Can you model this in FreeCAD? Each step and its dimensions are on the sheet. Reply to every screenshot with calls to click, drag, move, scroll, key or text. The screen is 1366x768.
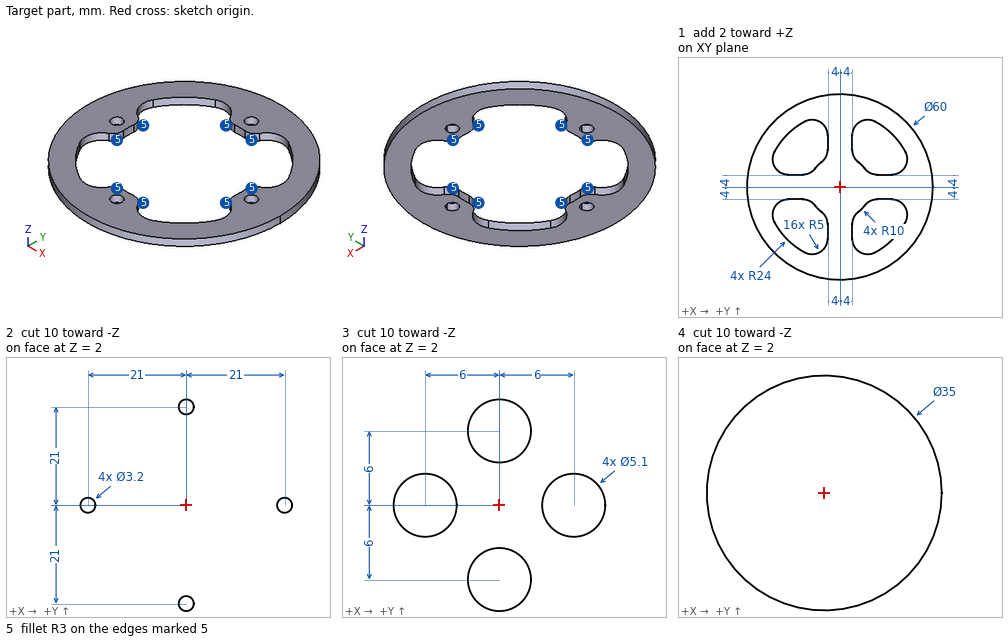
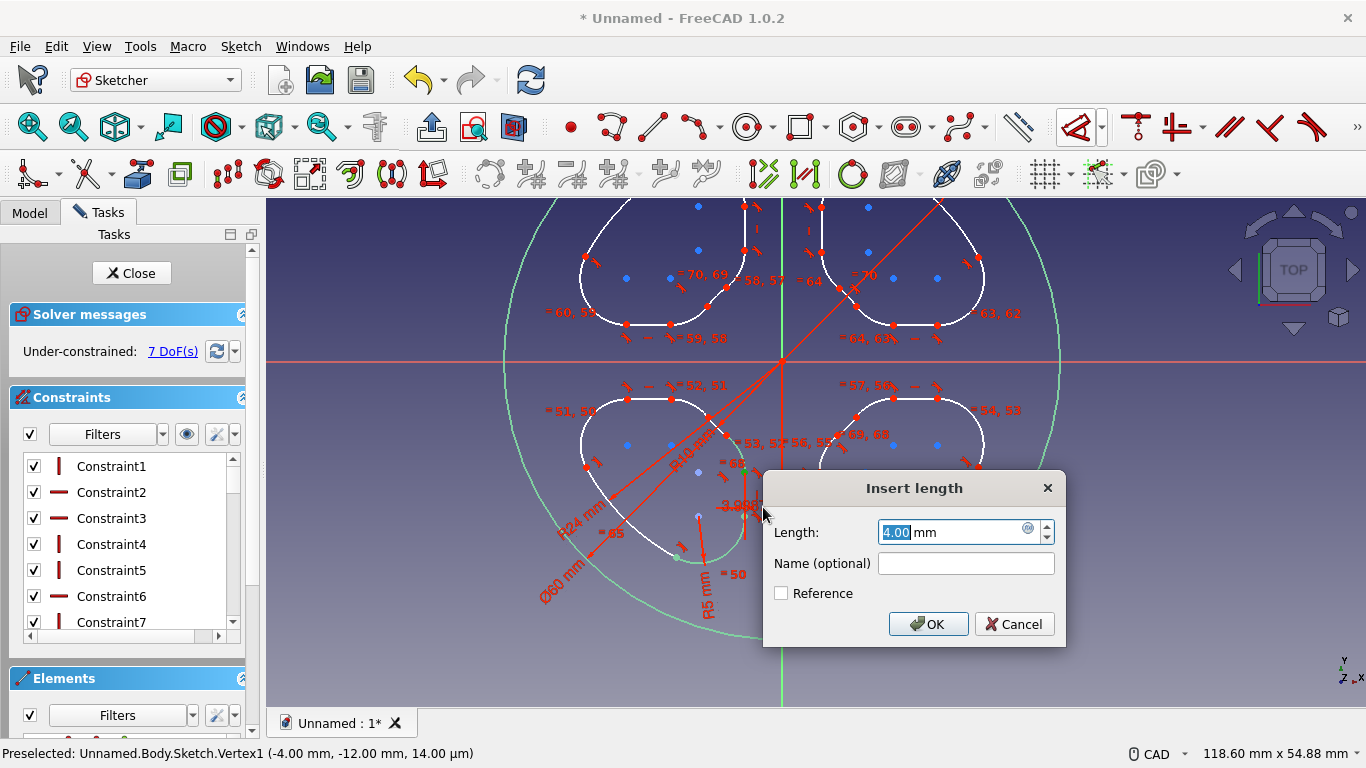
text(4)
key(Return)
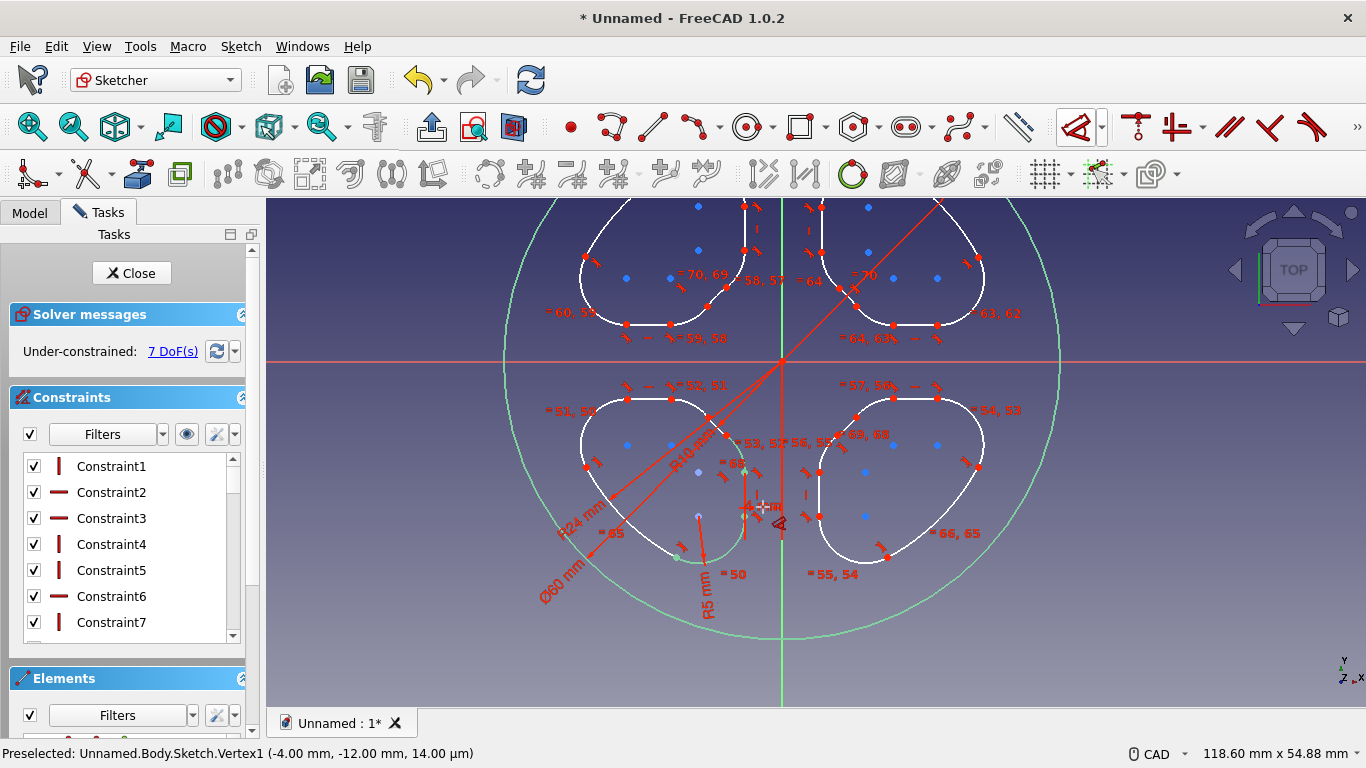
click(627, 399)
click(593, 380)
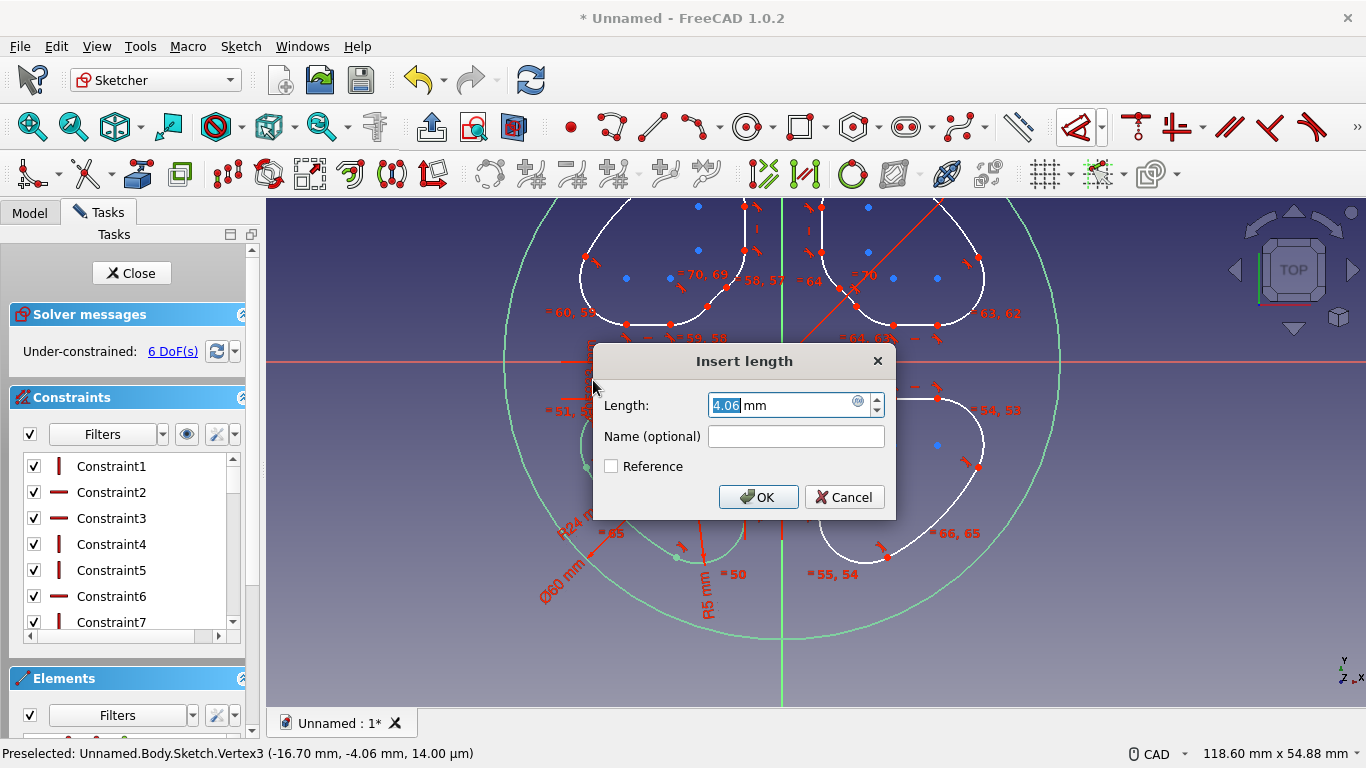
text(4)
key(Return)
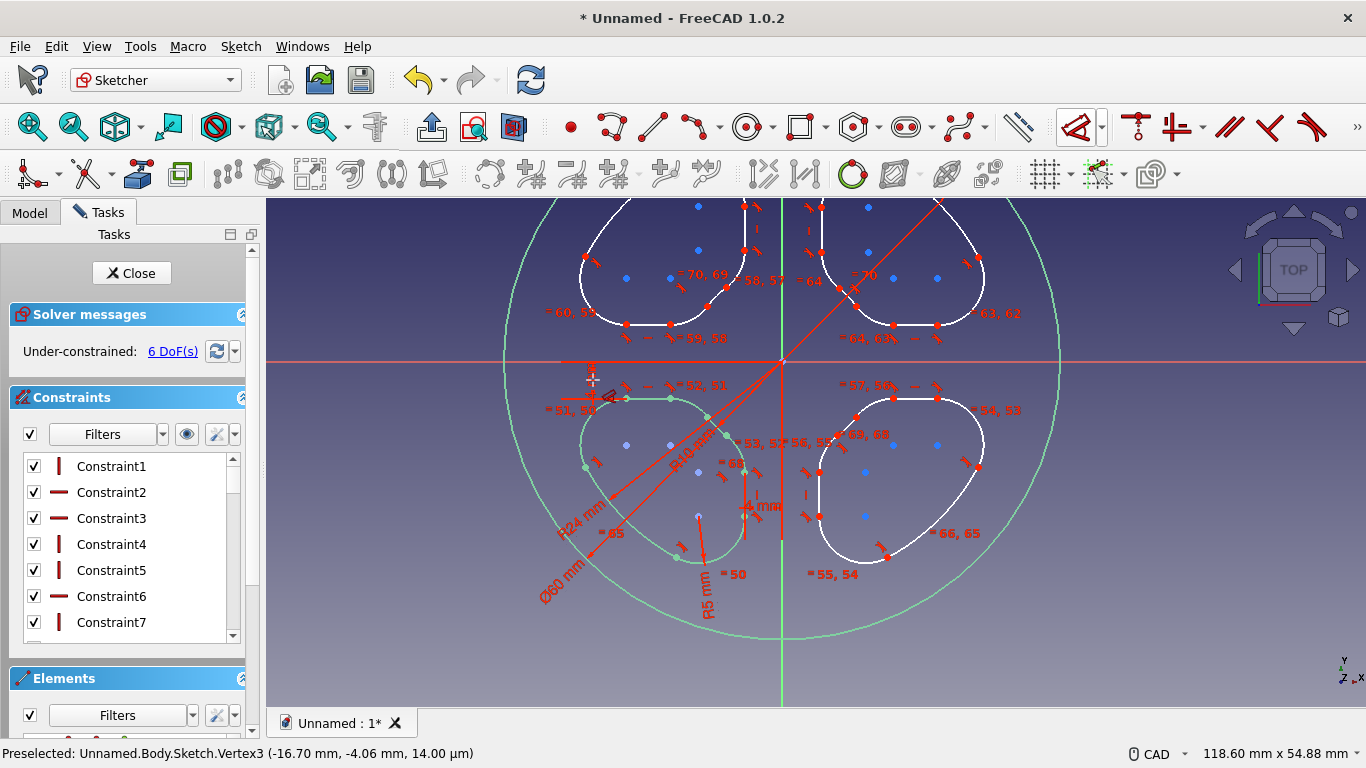
click(893, 399)
click(927, 380)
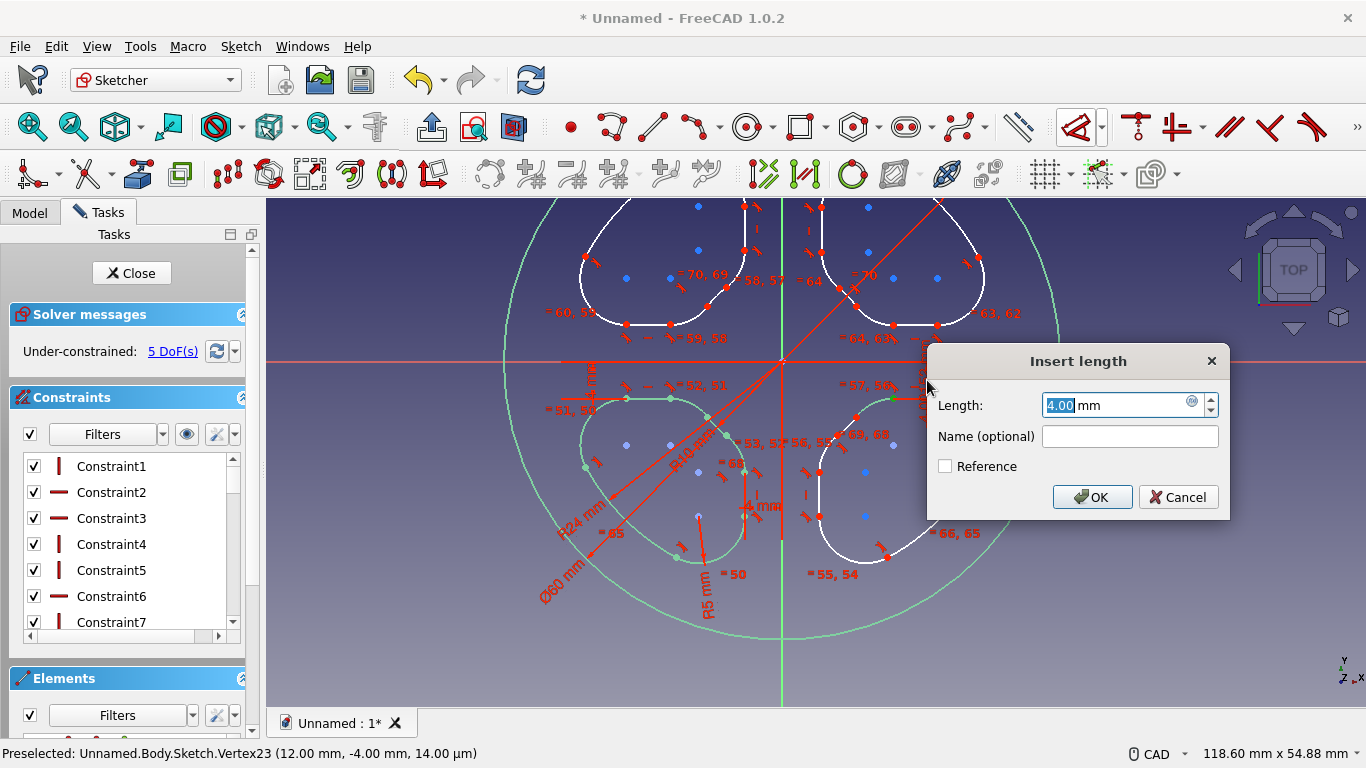
text(4)
key(Return)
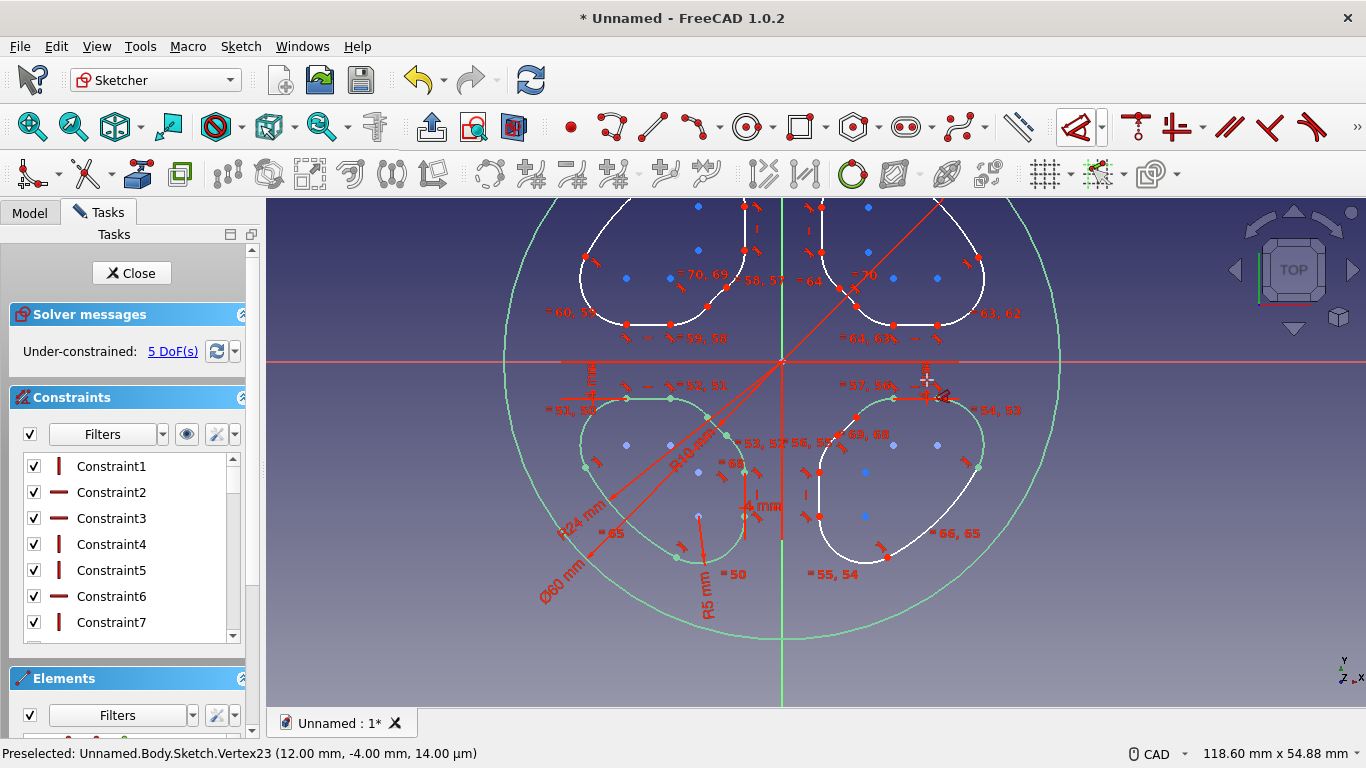
click(819, 517)
click(801, 551)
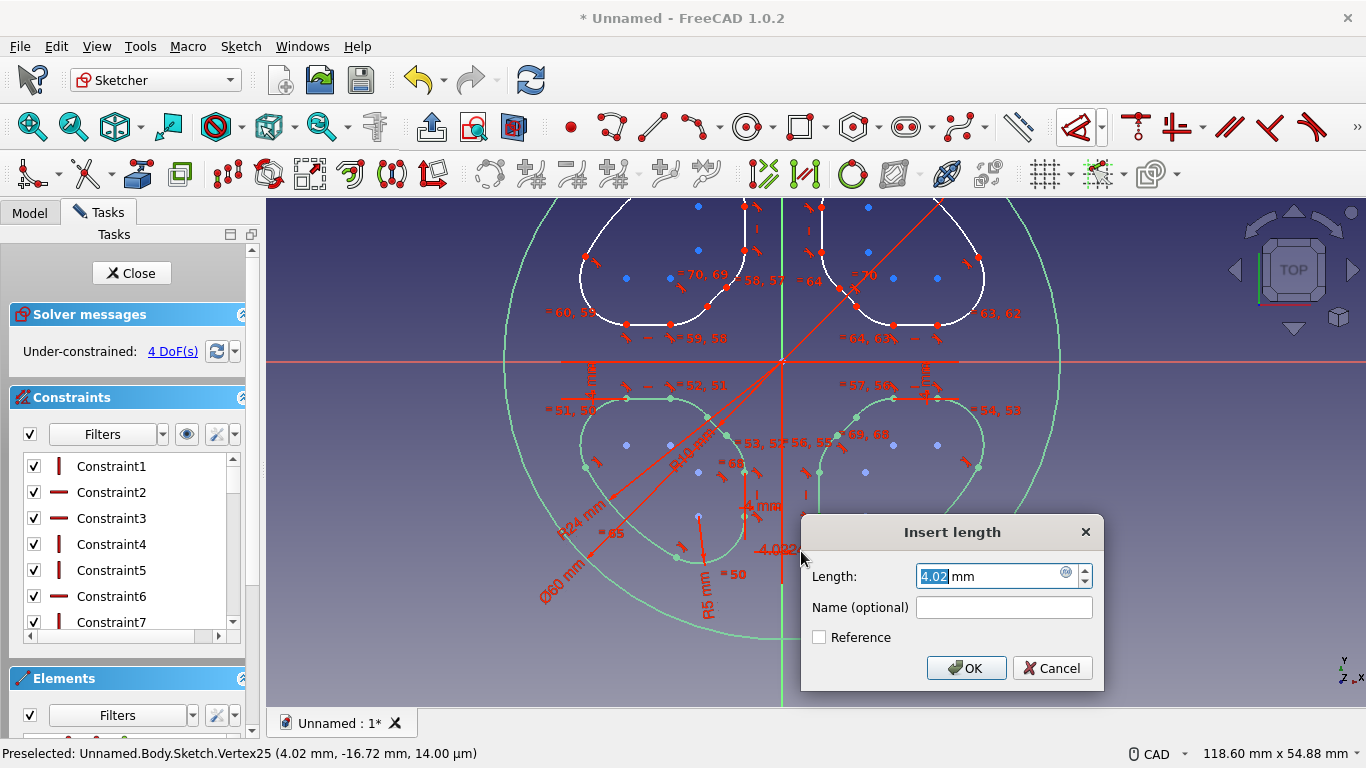
text(4)
key(Return)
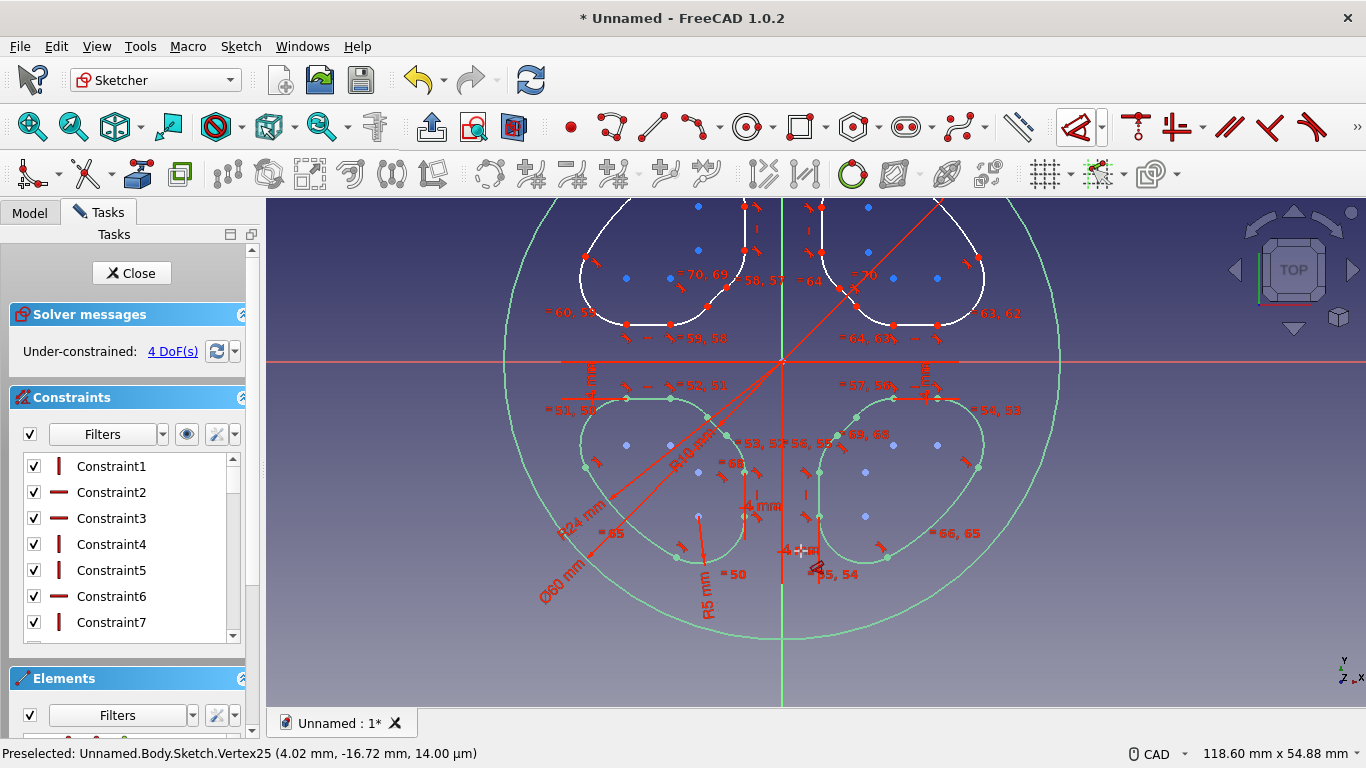
scroll(705, 563, down, 3)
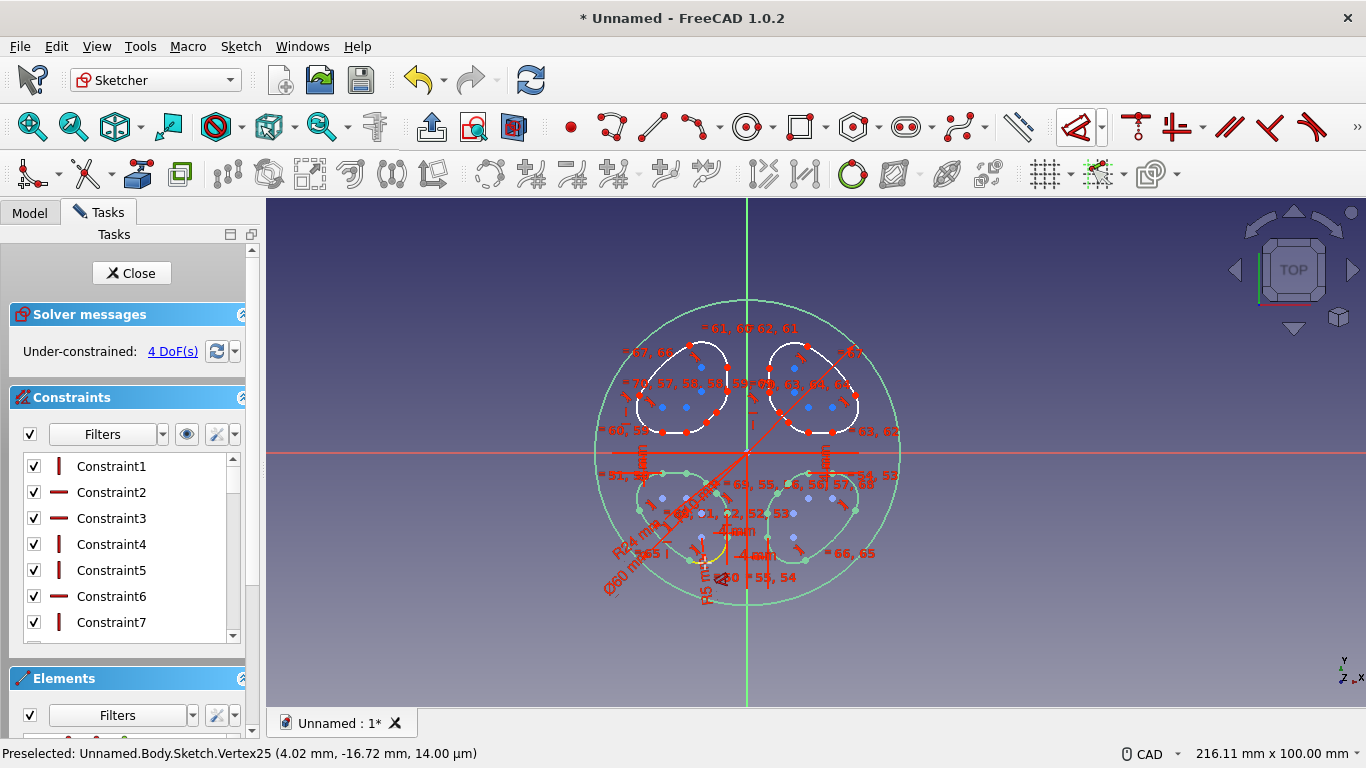
scroll(727, 368, up, 4)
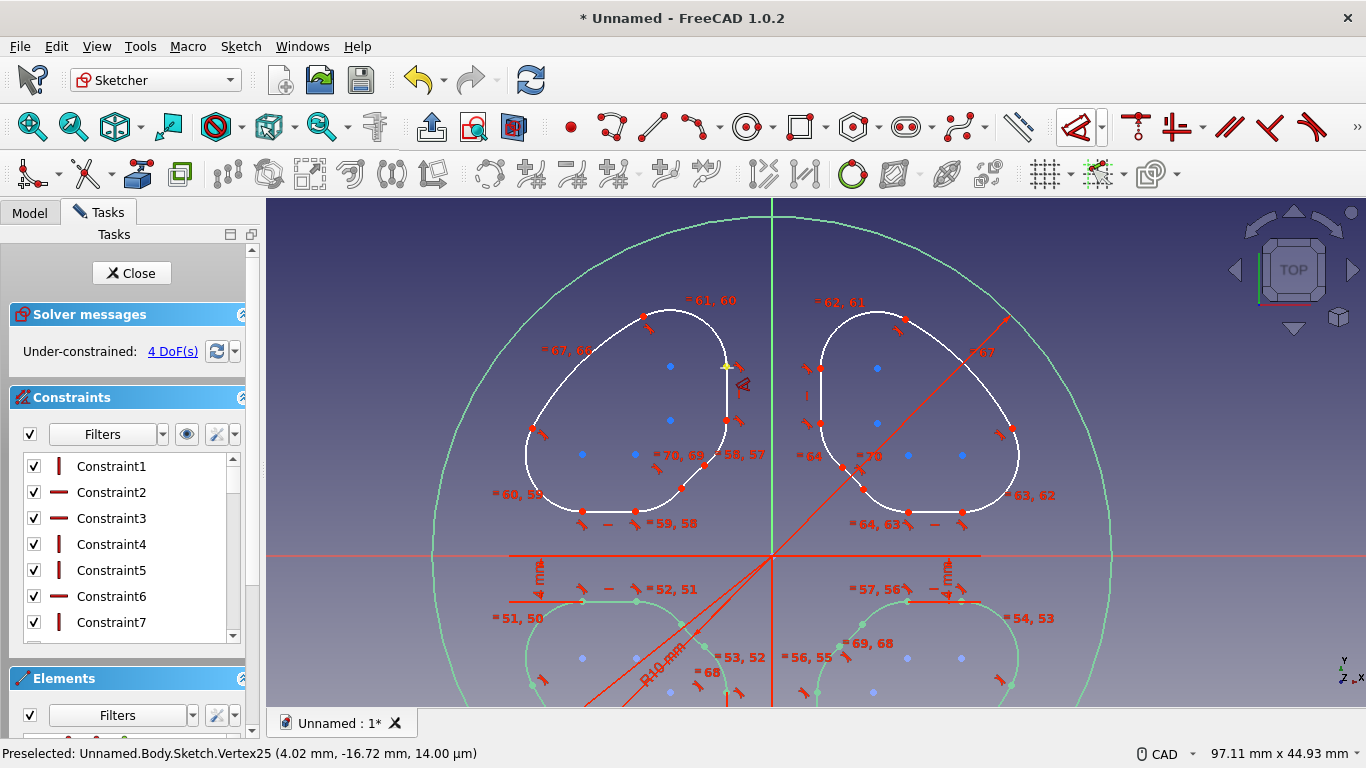
click(727, 367)
click(749, 333)